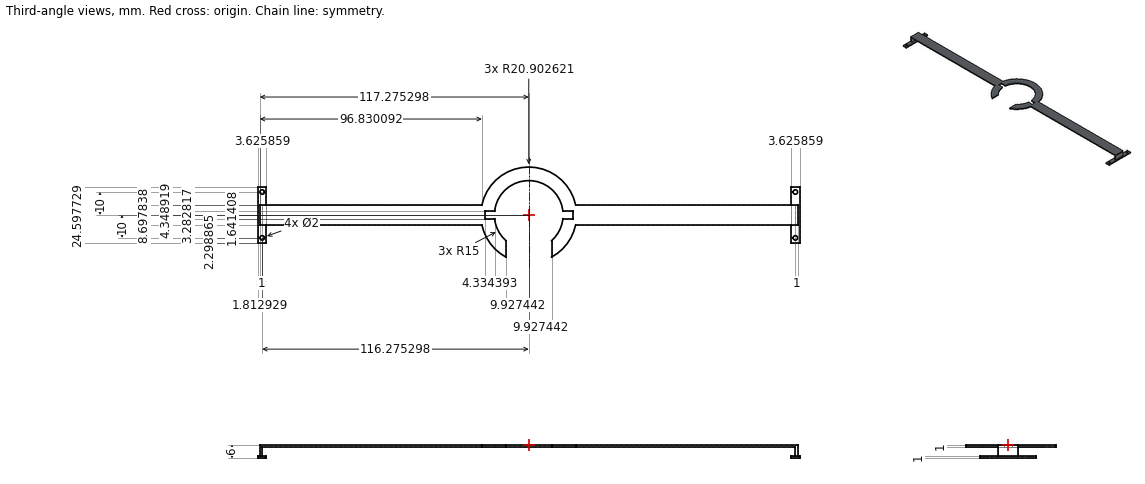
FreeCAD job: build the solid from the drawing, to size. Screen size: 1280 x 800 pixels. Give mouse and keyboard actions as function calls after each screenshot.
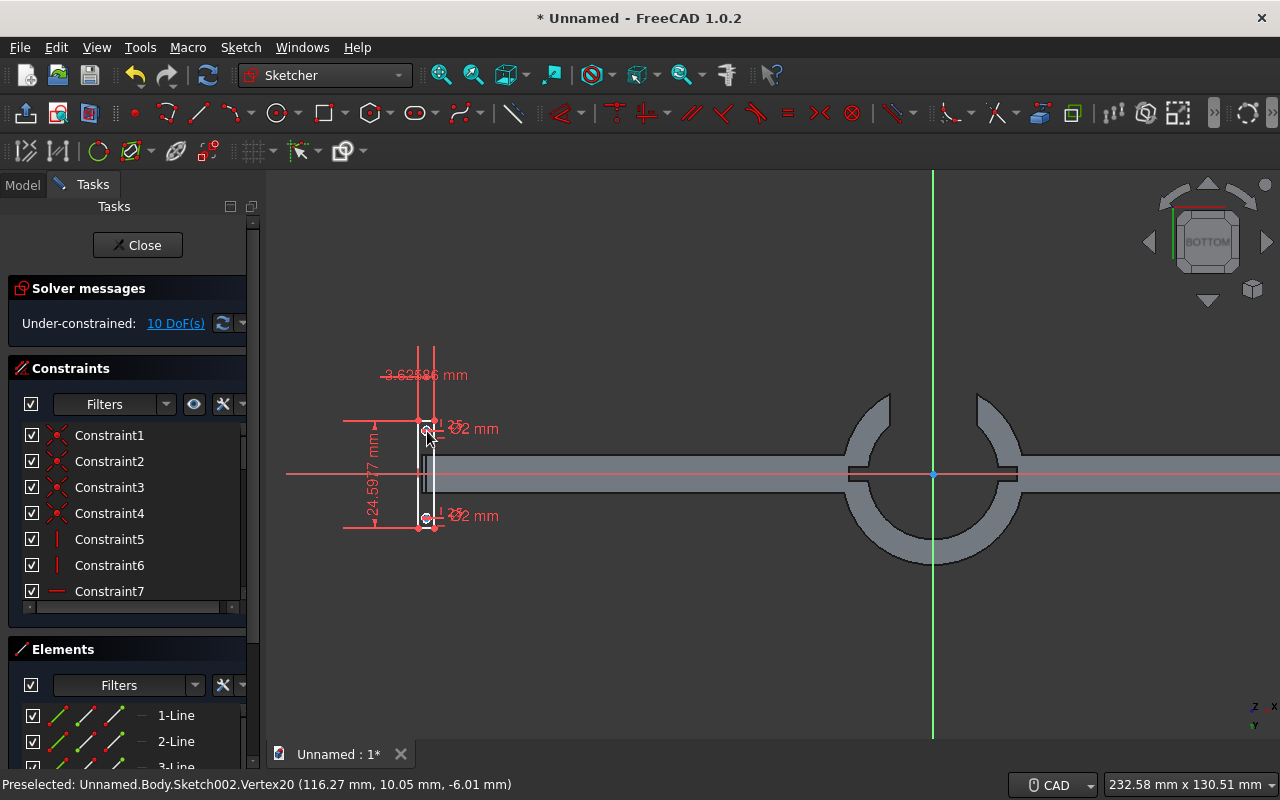
click(426, 431)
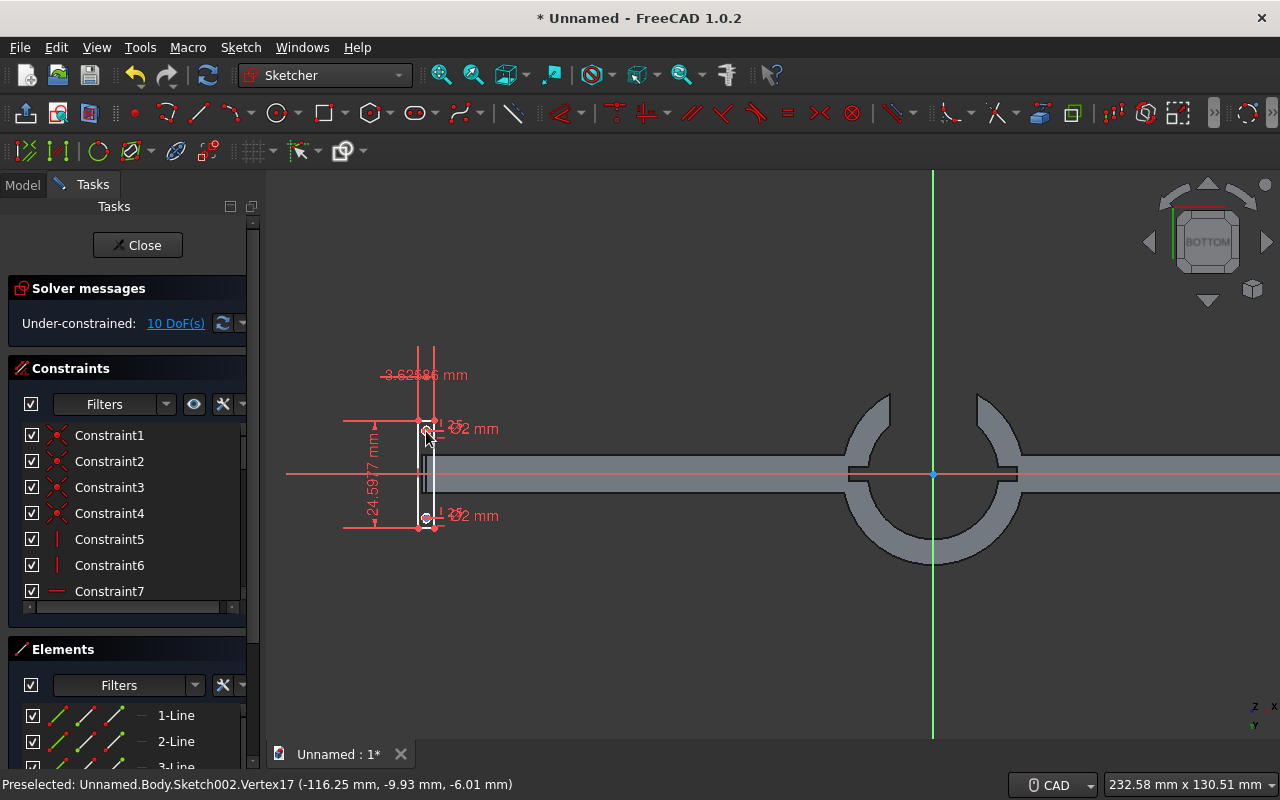
scroll(426, 431, down, 3)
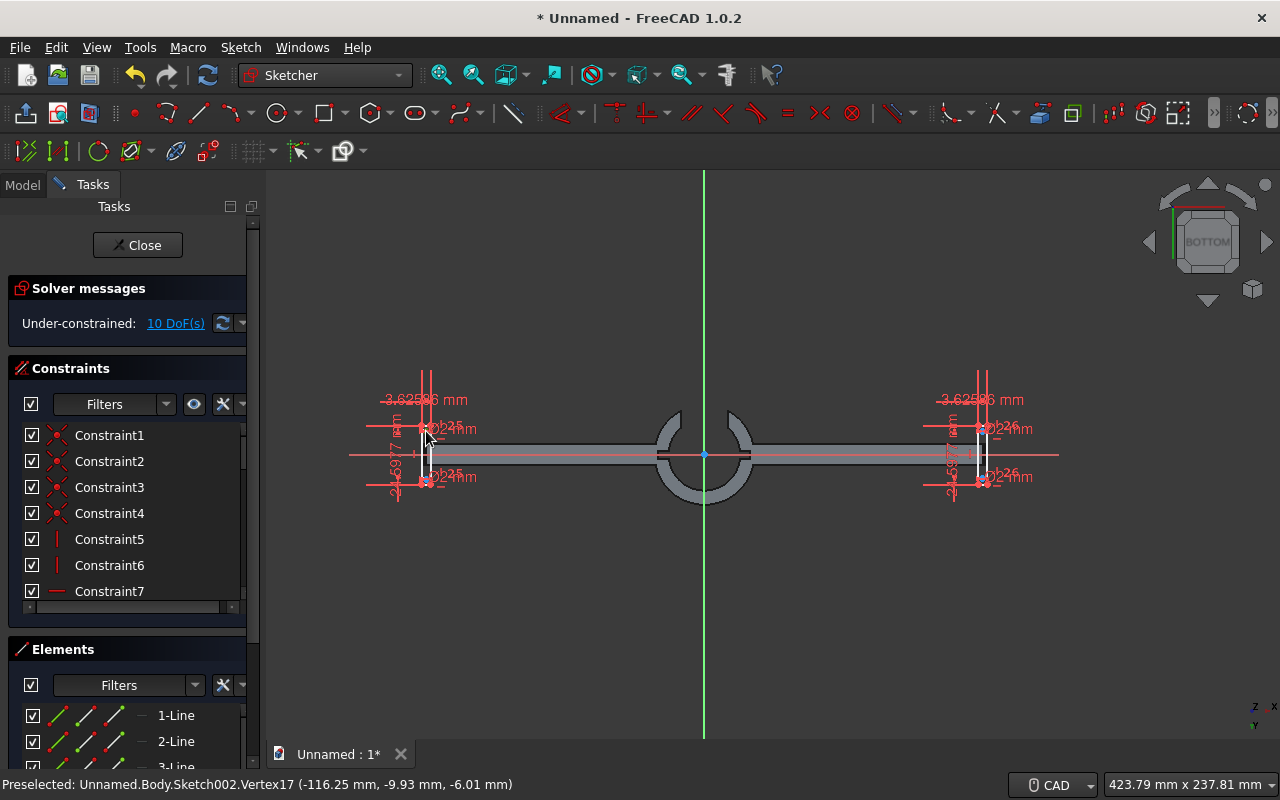
scroll(983, 431, up, 3)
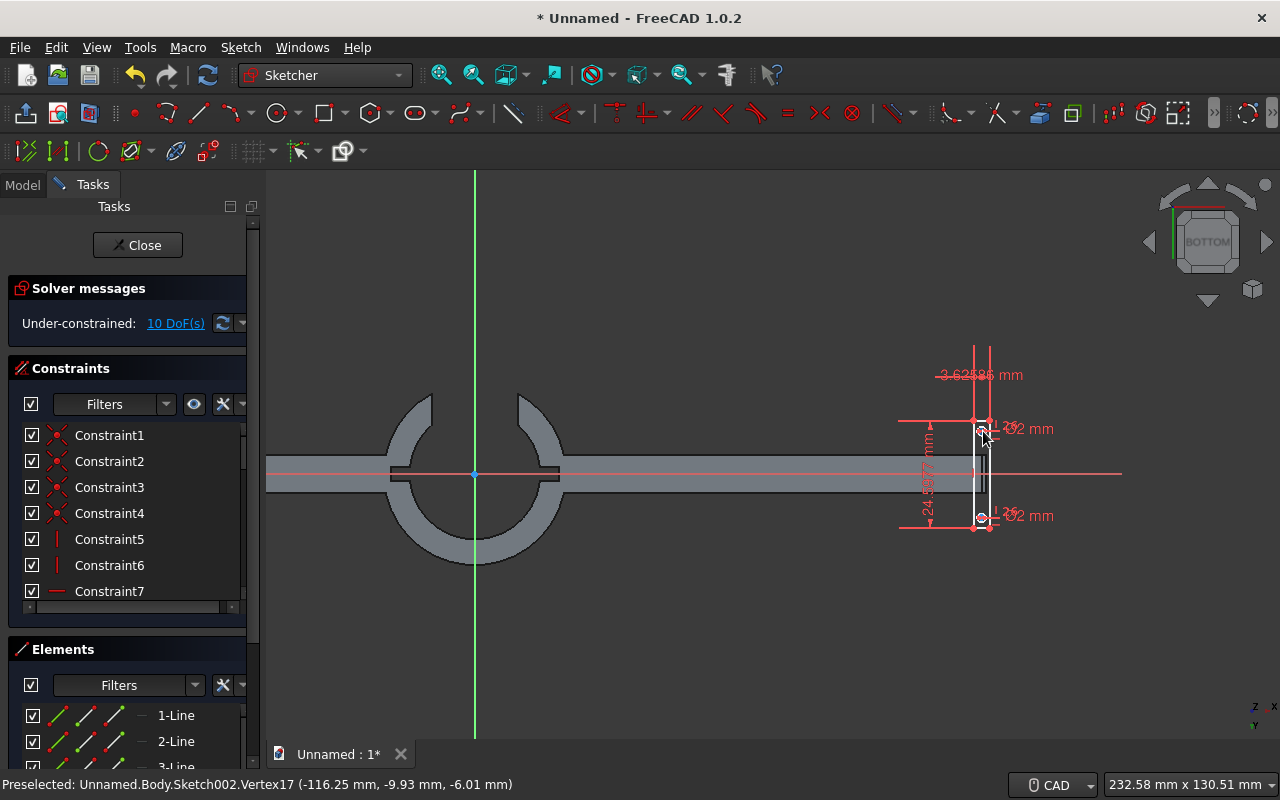
click(982, 431)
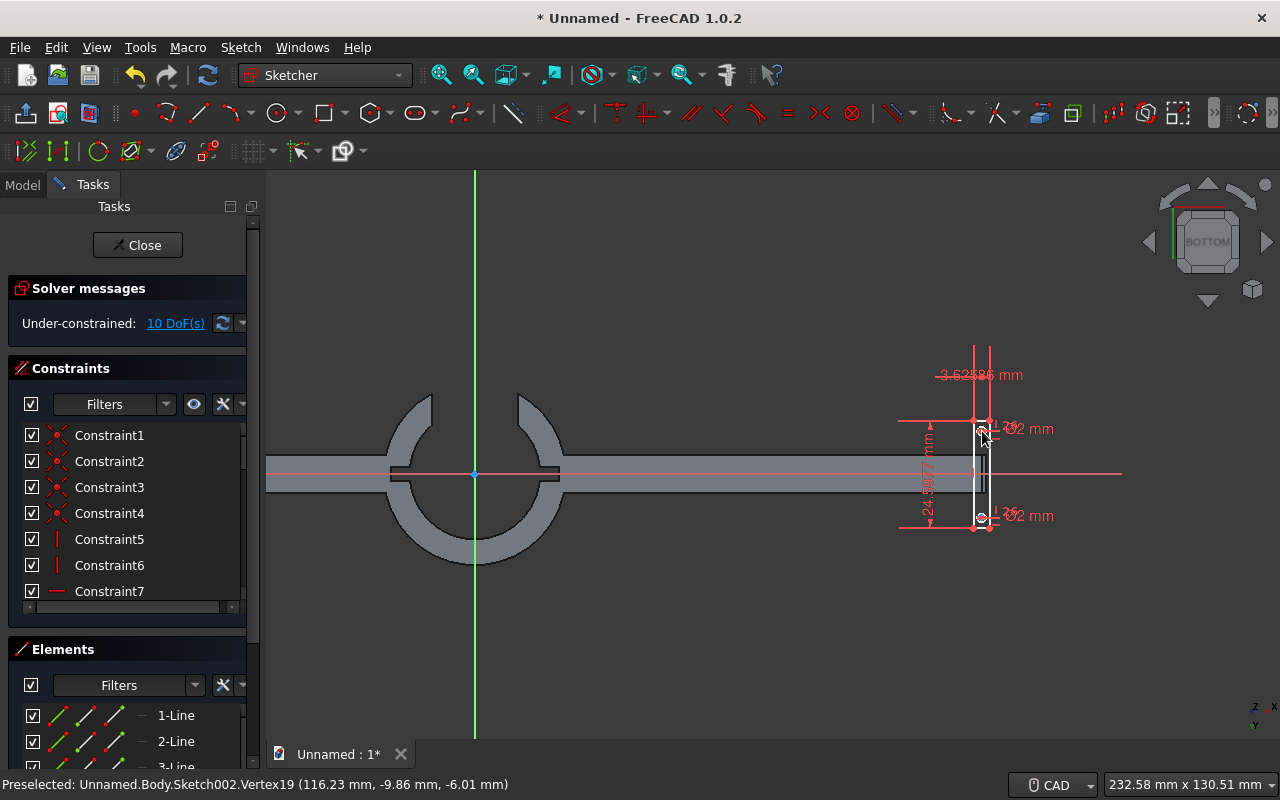
click(475, 674)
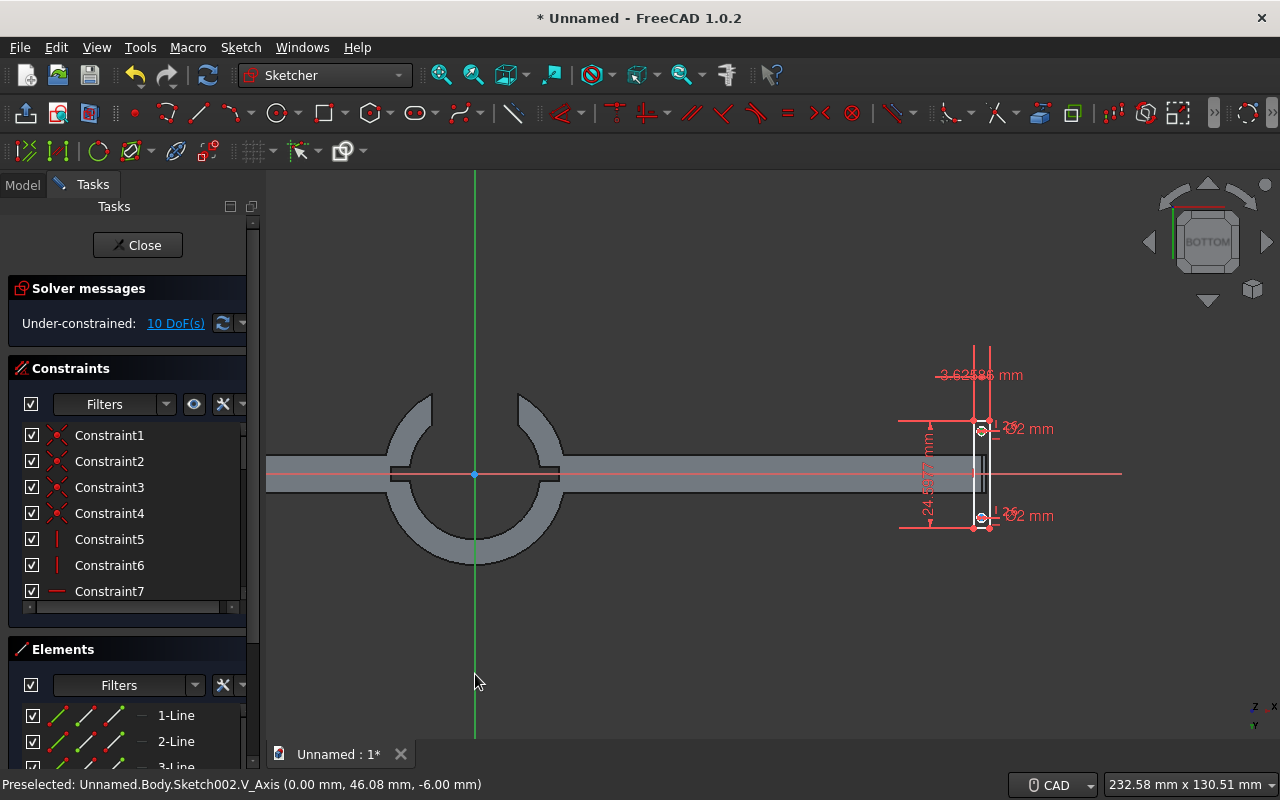
click(820, 114)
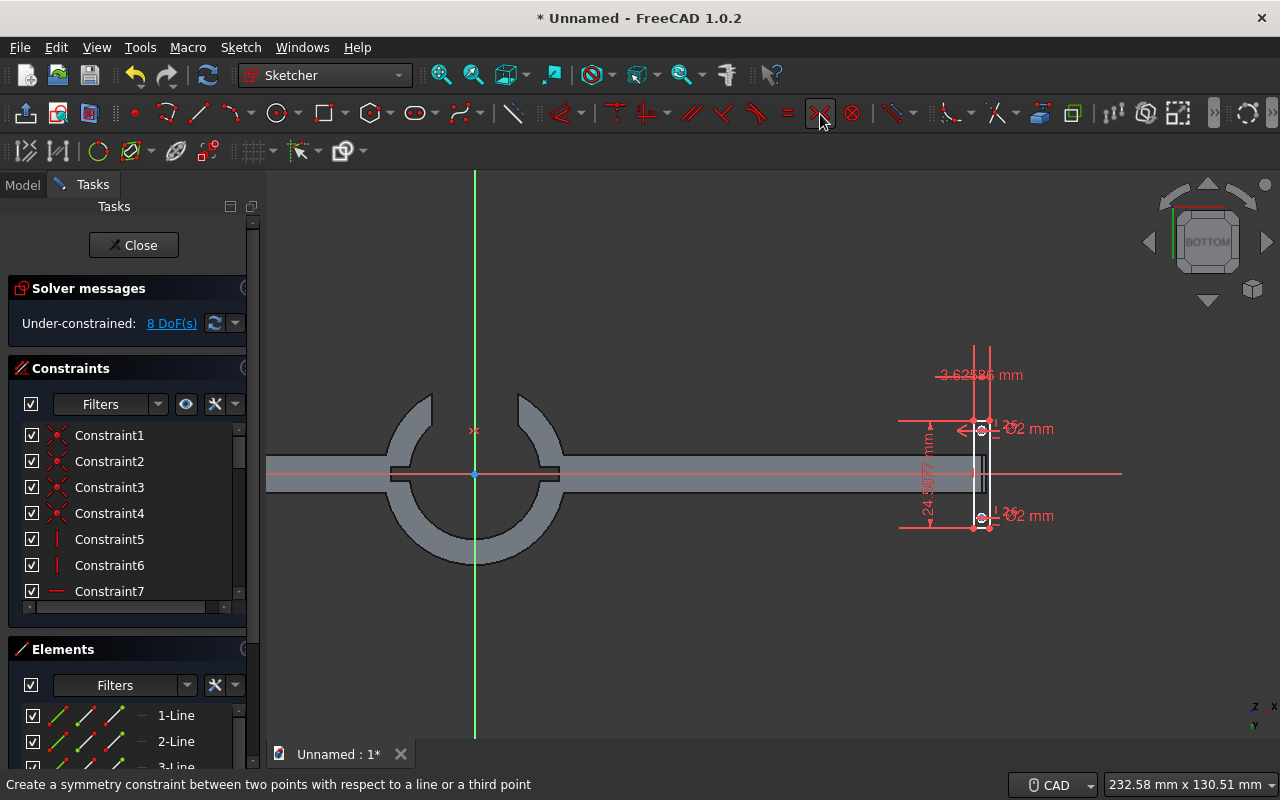
scroll(984, 431, down, 3)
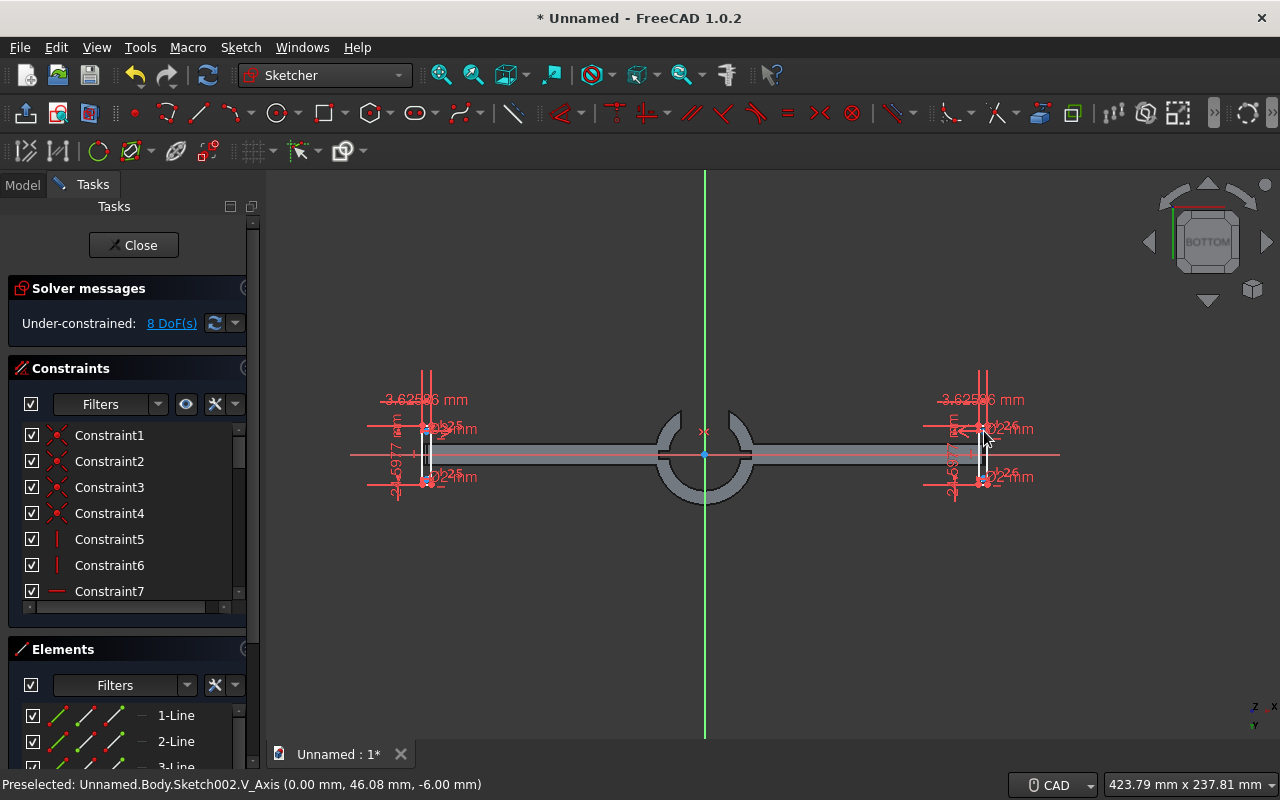
scroll(431, 426, up, 3)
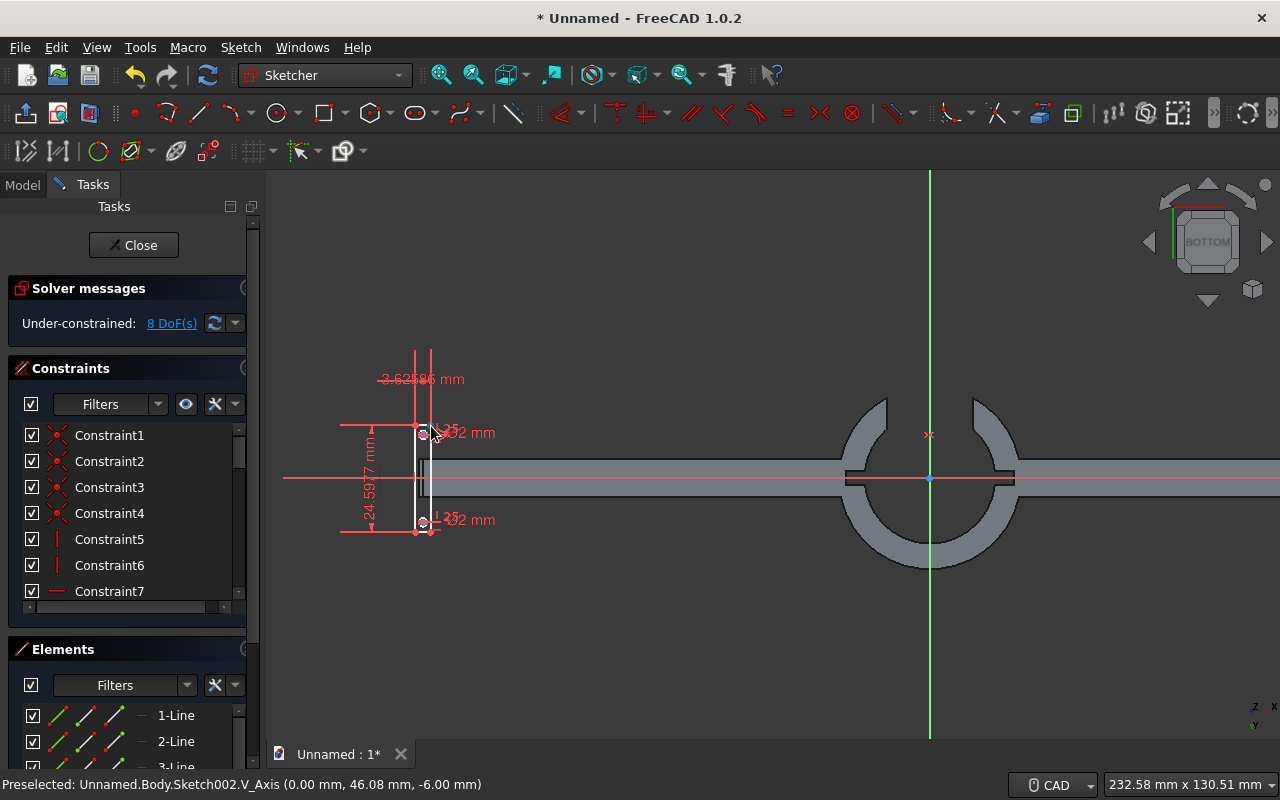
click(431, 425)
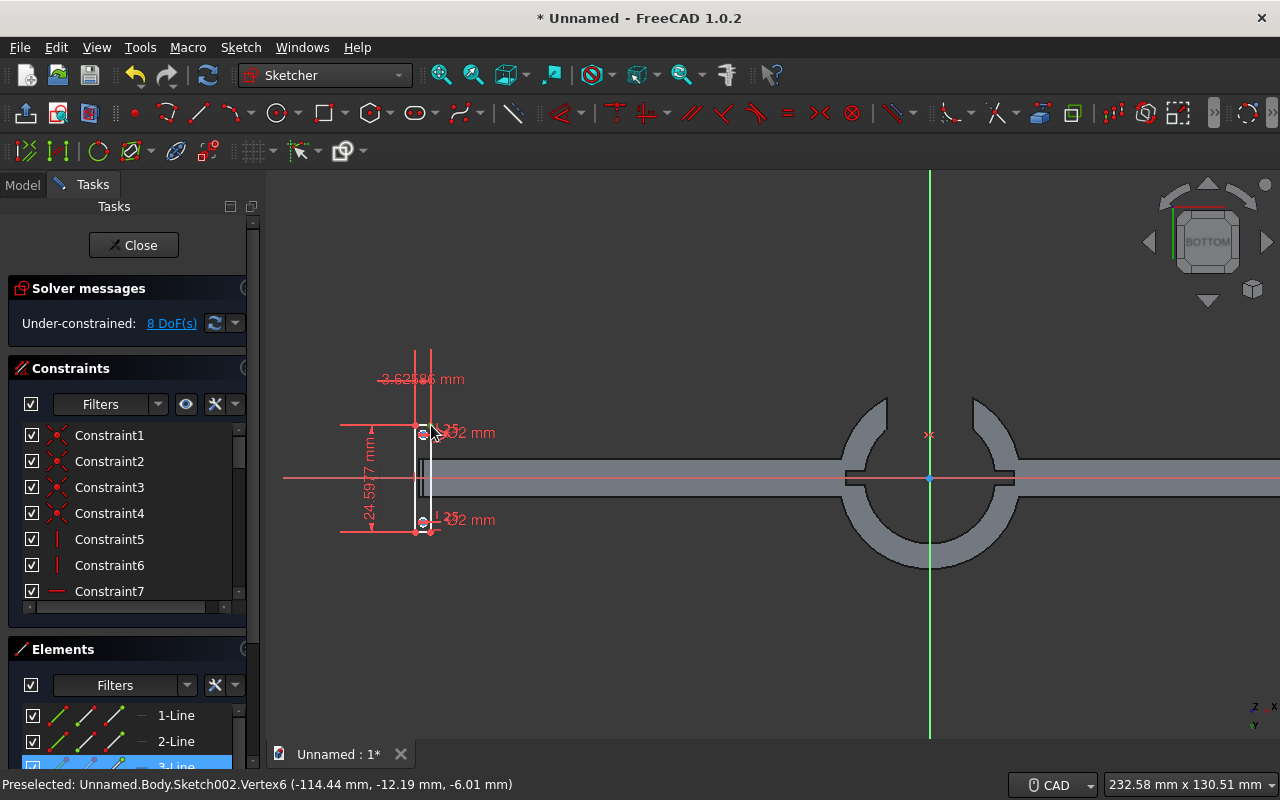
scroll(430, 426, down, 3)